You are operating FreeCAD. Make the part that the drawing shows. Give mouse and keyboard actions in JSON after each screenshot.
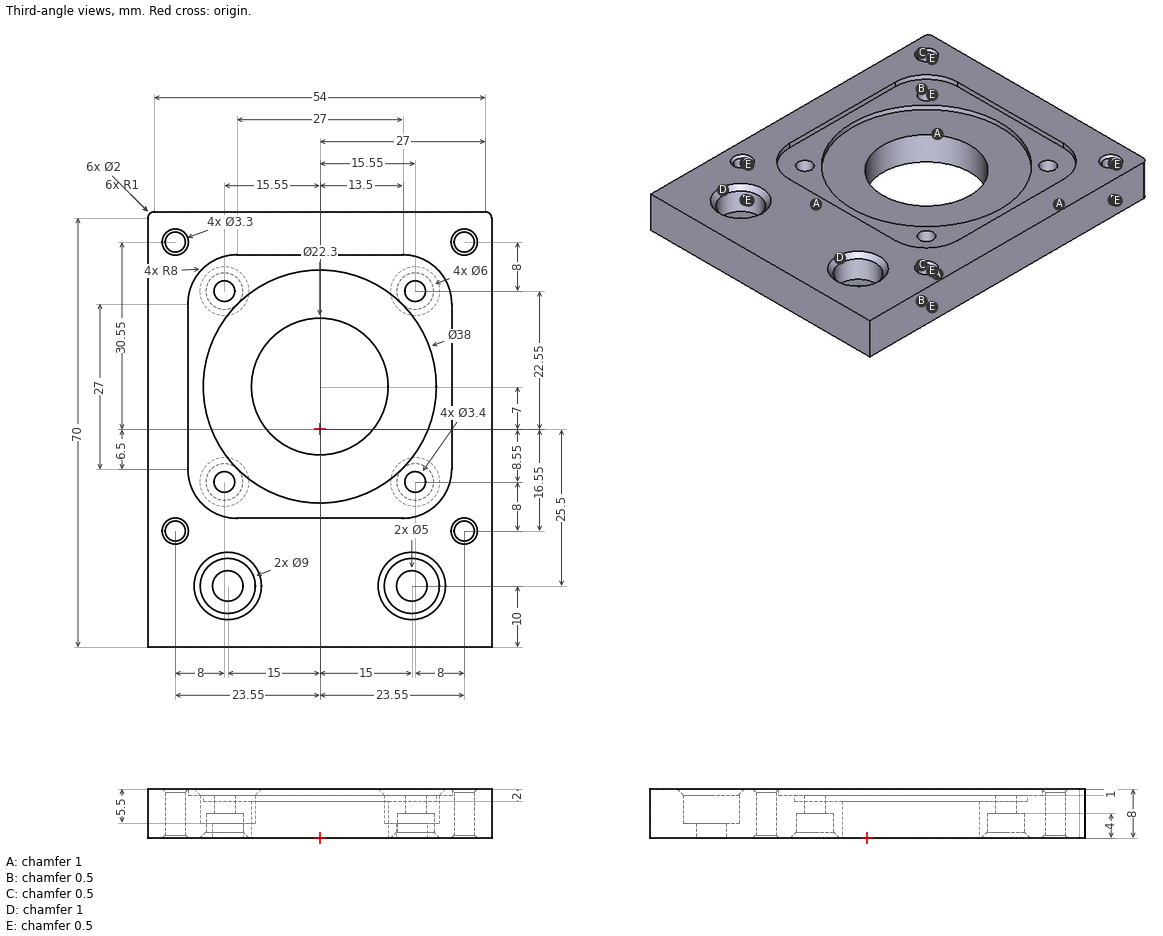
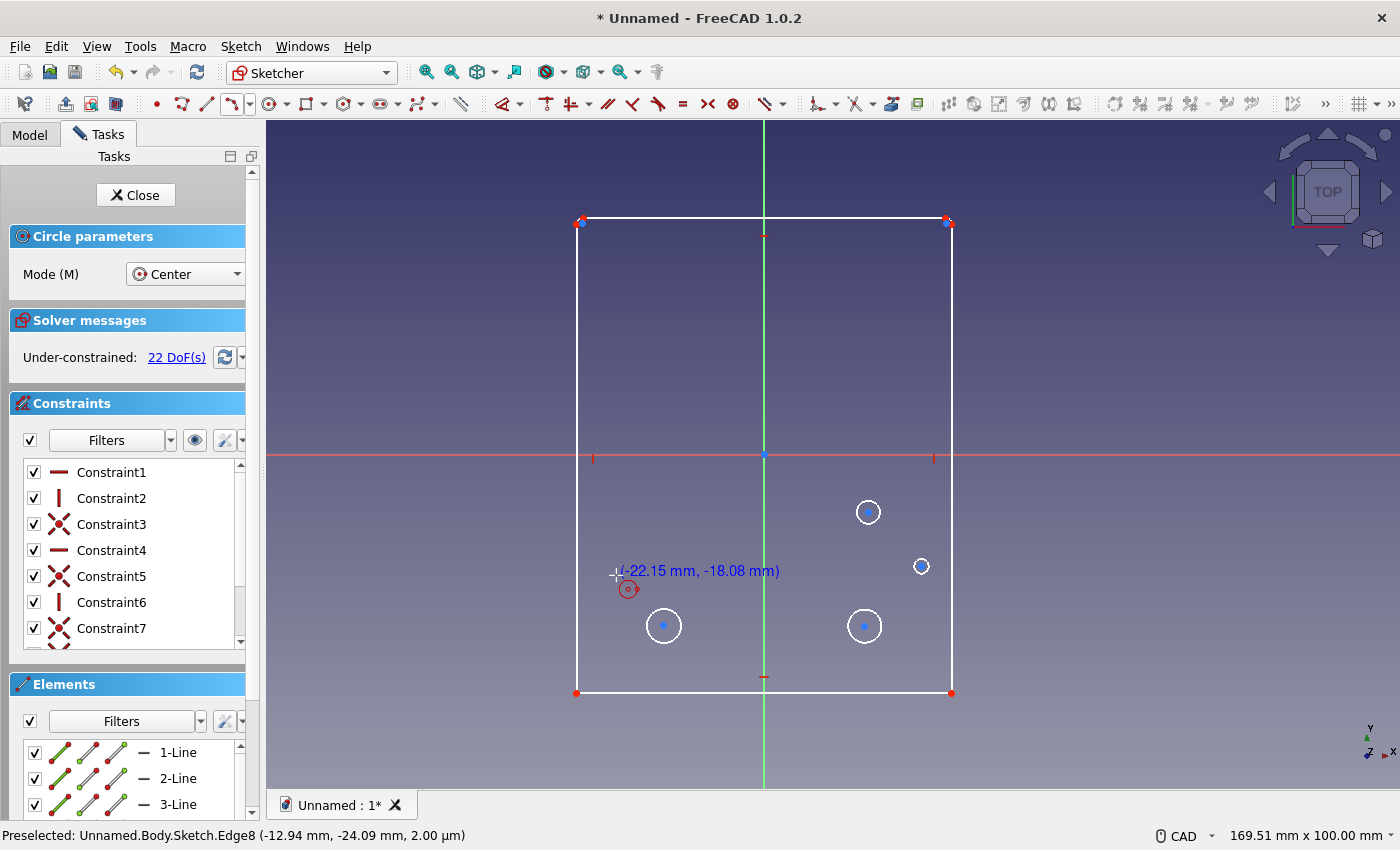
{"action": "left_click", "coordinate": [607, 566]}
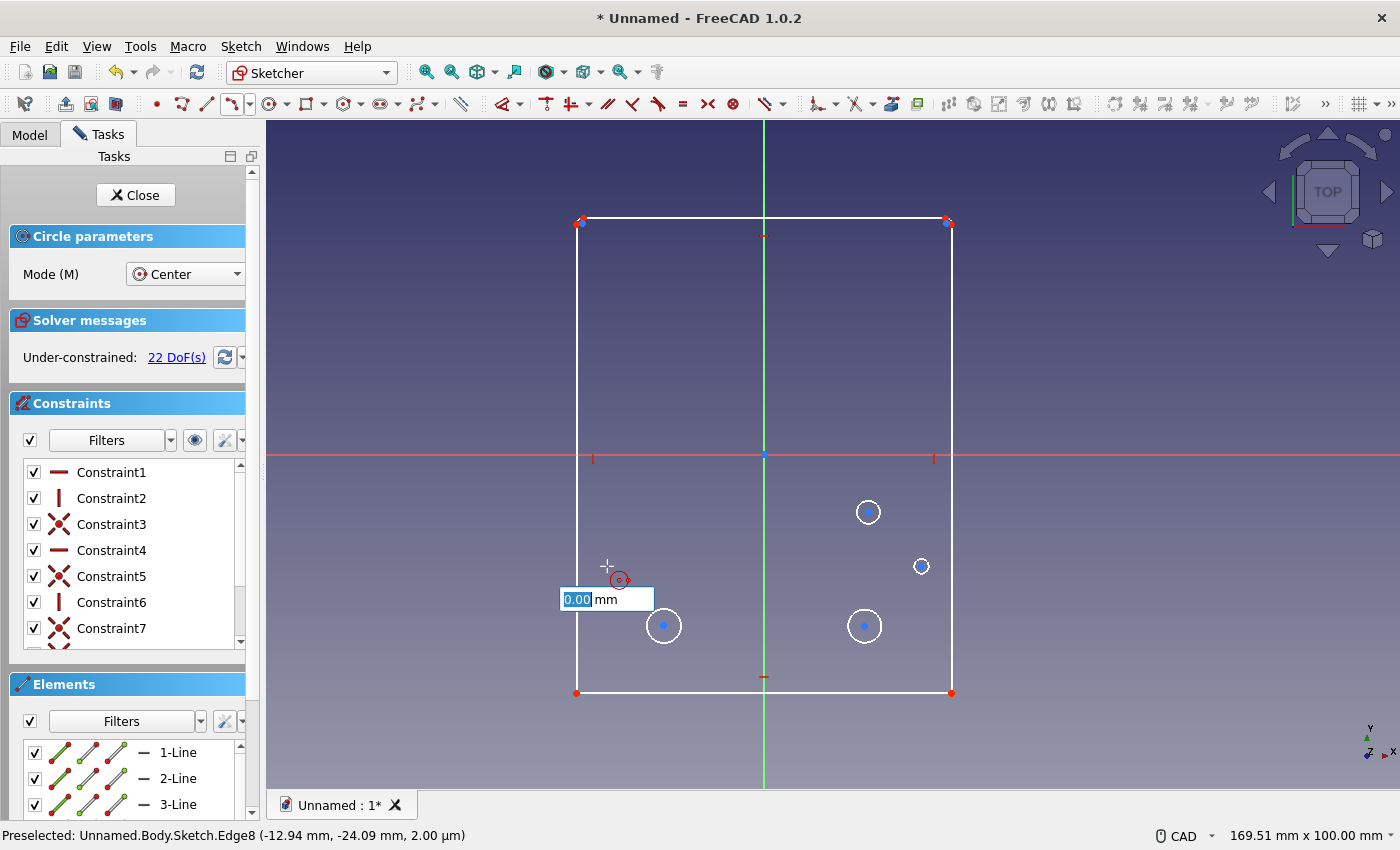
{"action": "scroll", "coordinate": [612, 561], "scroll_direction": "up", "scroll_amount": 5}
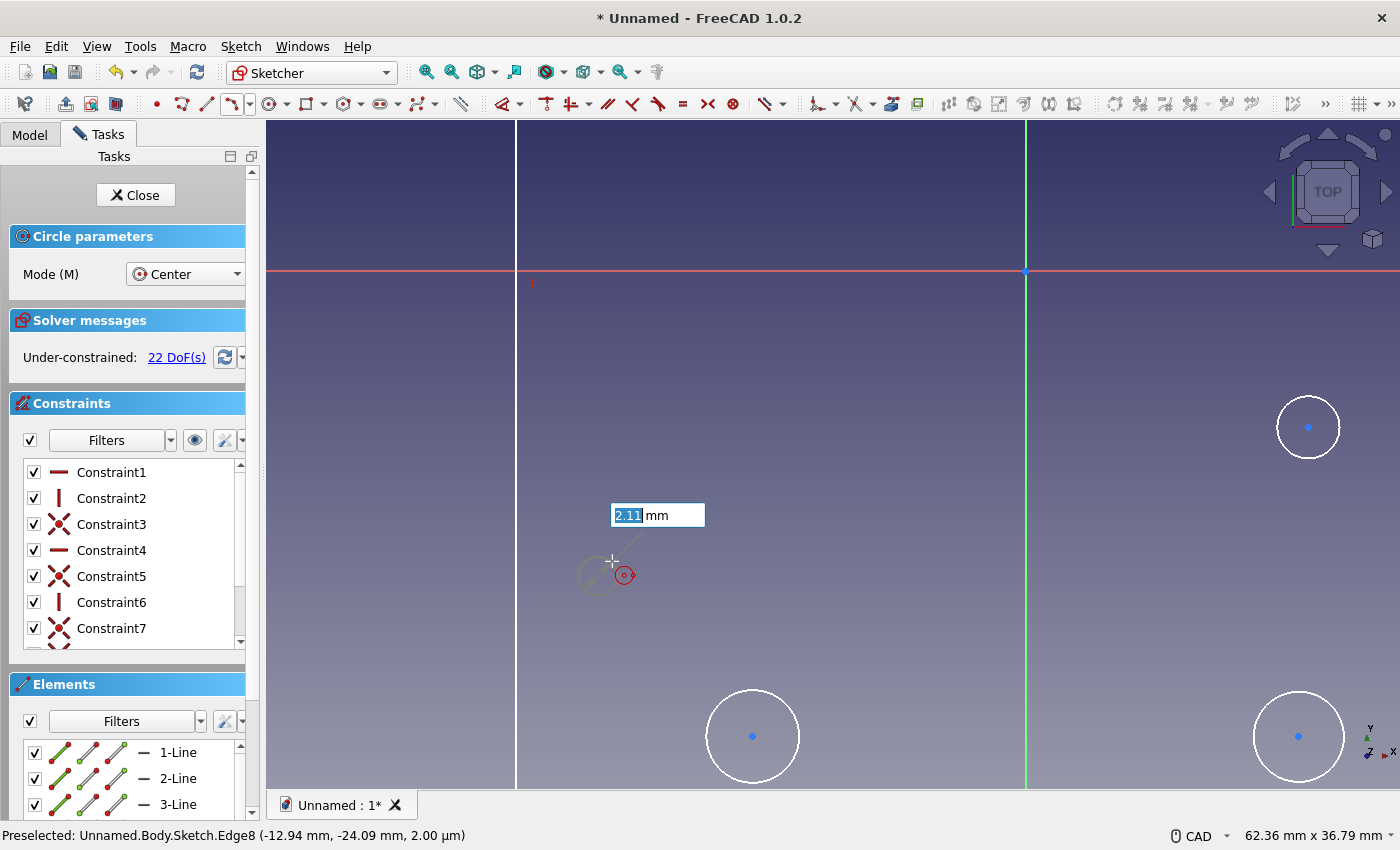
{"action": "left_click", "coordinate": [610, 559]}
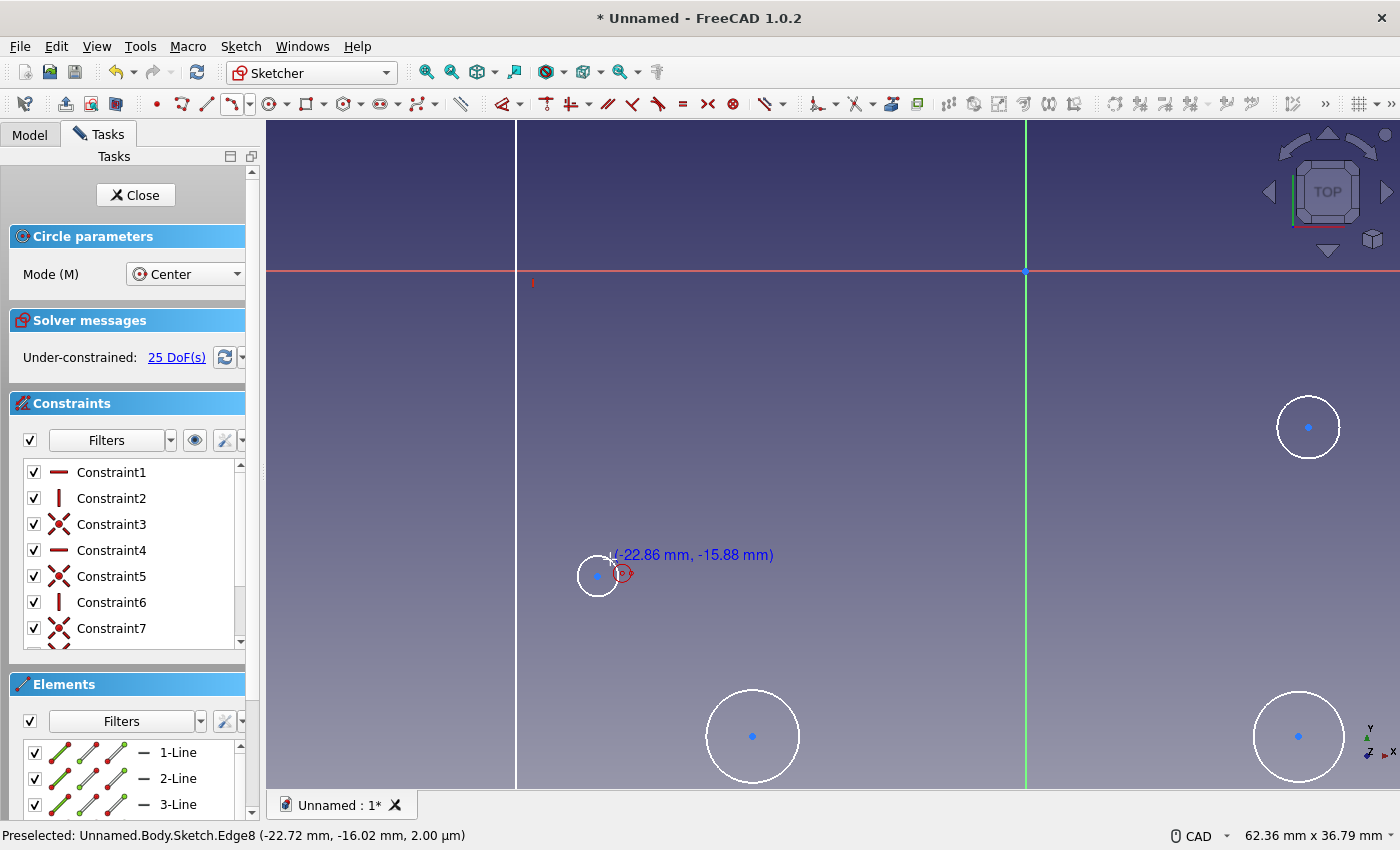
{"action": "left_click", "coordinate": [743, 427]}
{"action": "left_click", "coordinate": [765, 405]}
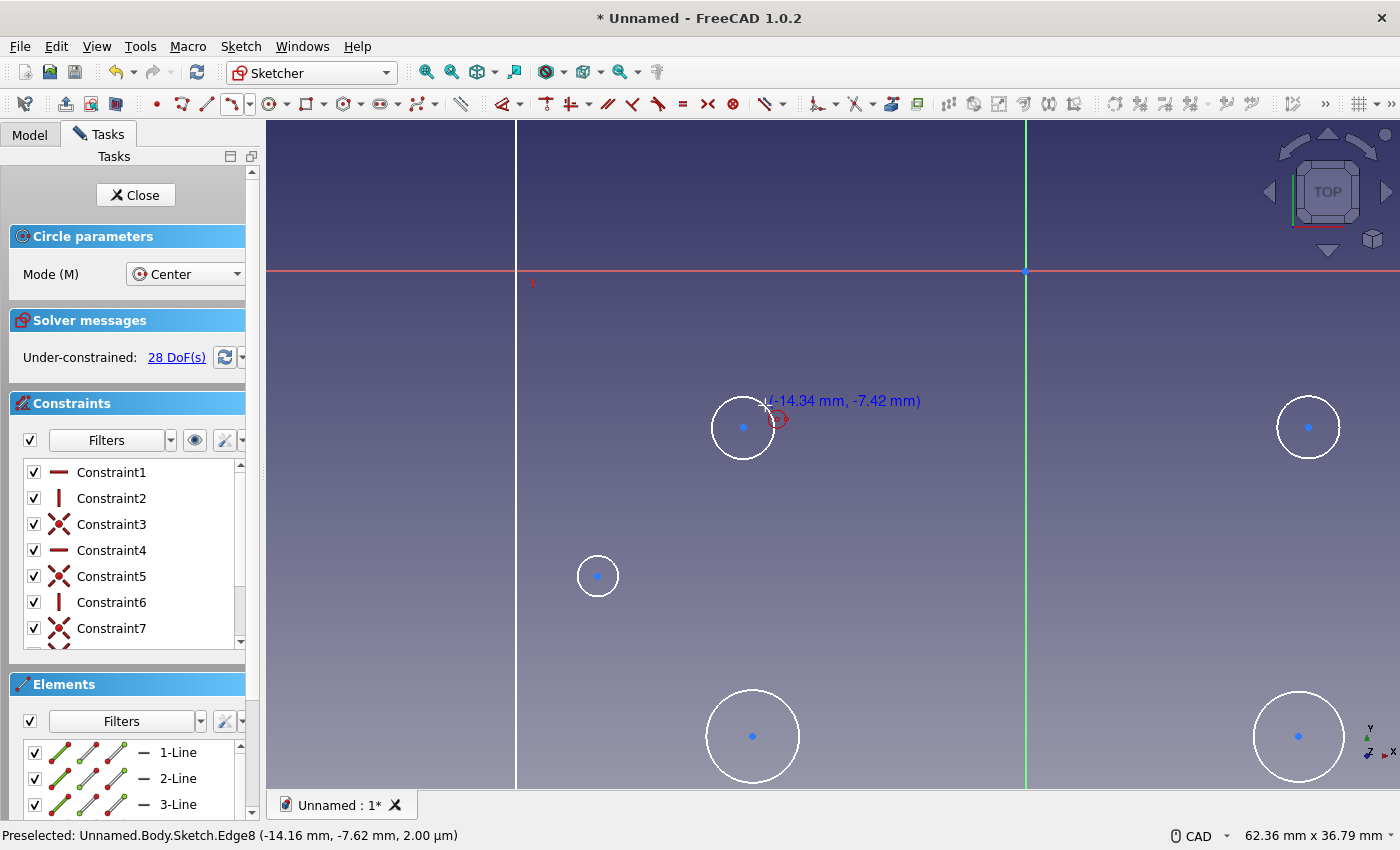
{"action": "scroll", "coordinate": [612, 561], "scroll_direction": "down", "scroll_amount": 5}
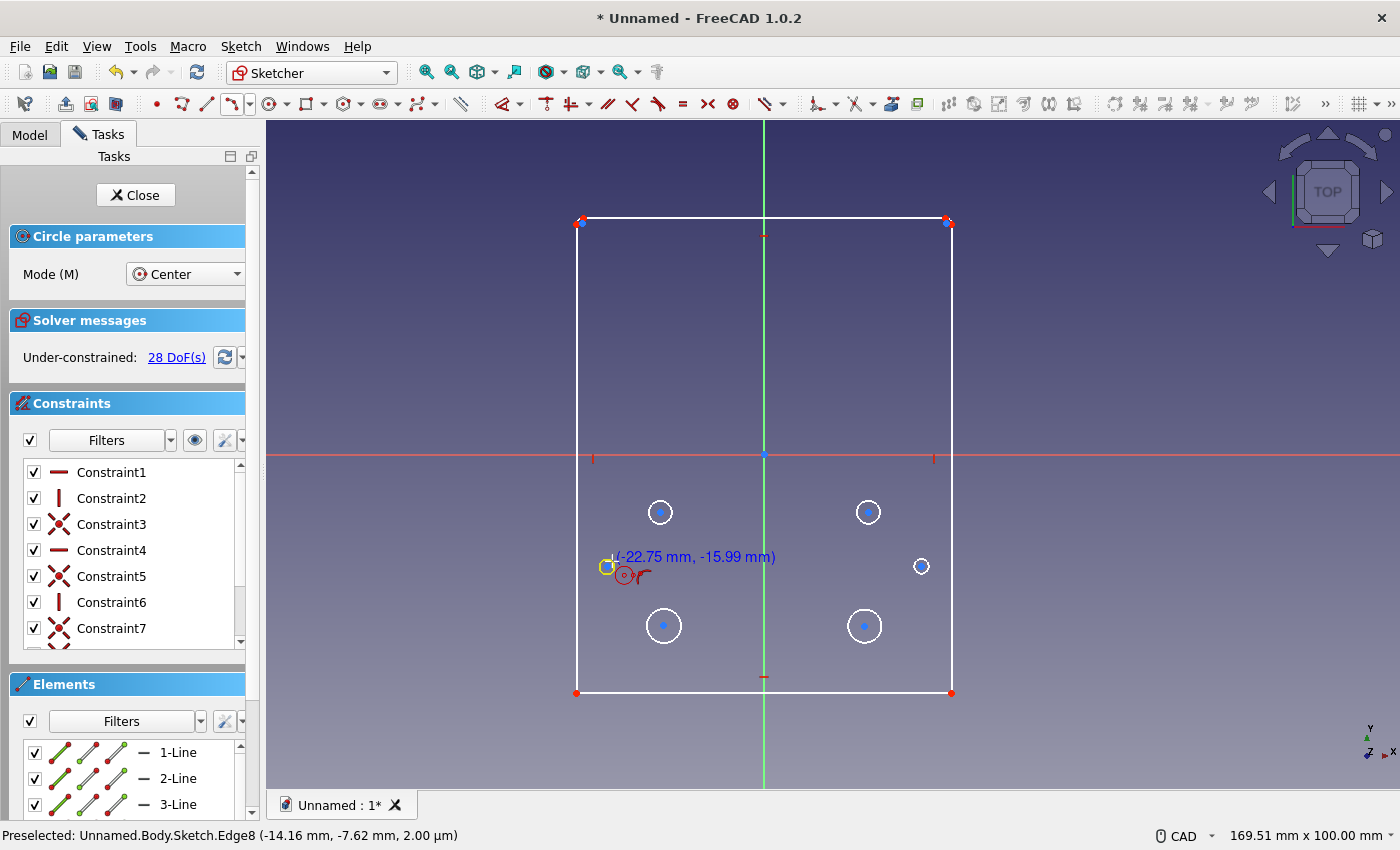
{"action": "scroll", "coordinate": [868, 304], "scroll_direction": "up", "scroll_amount": 4}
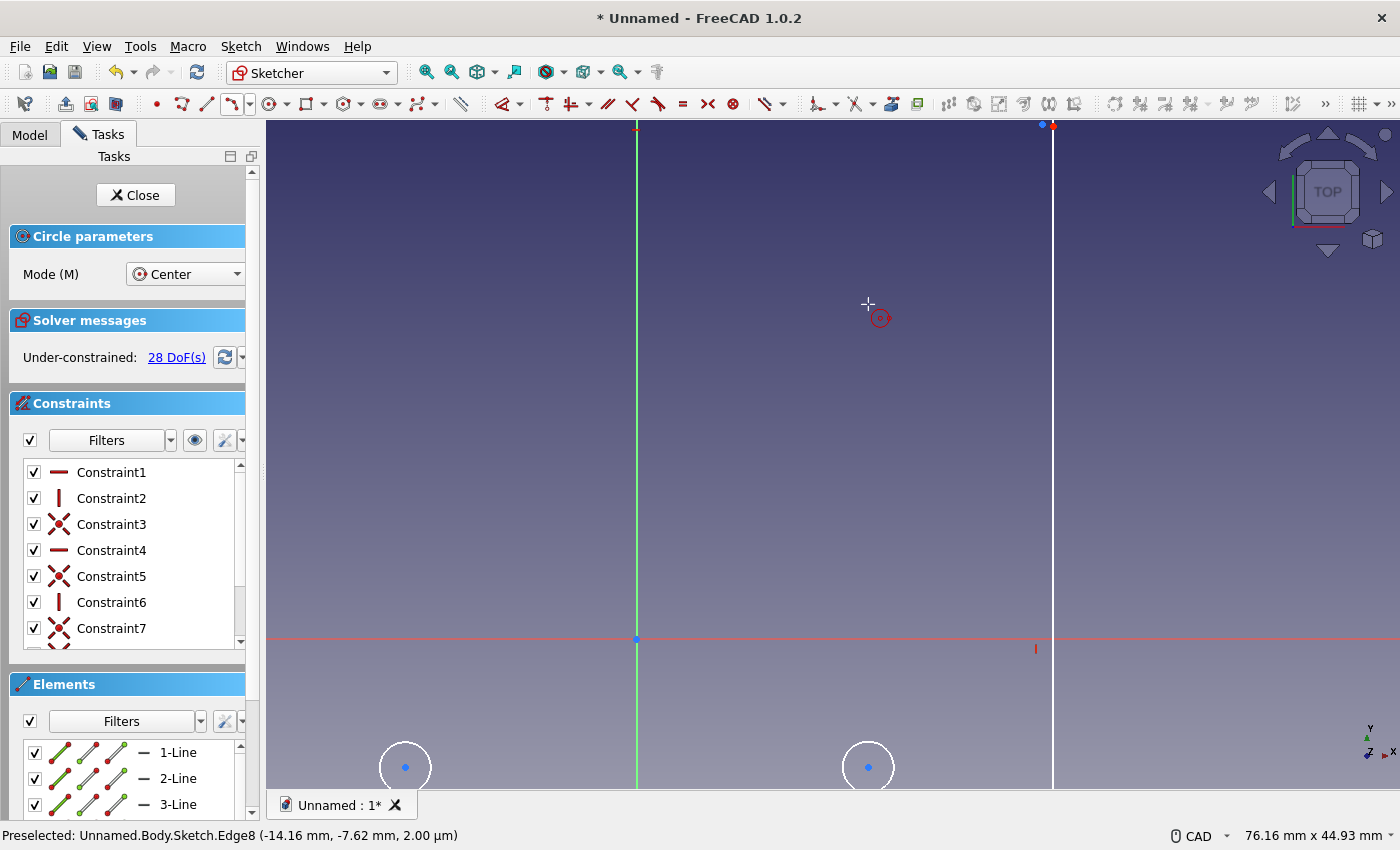
{"action": "left_click", "coordinate": [868, 303]}
{"action": "left_click", "coordinate": [886, 286]}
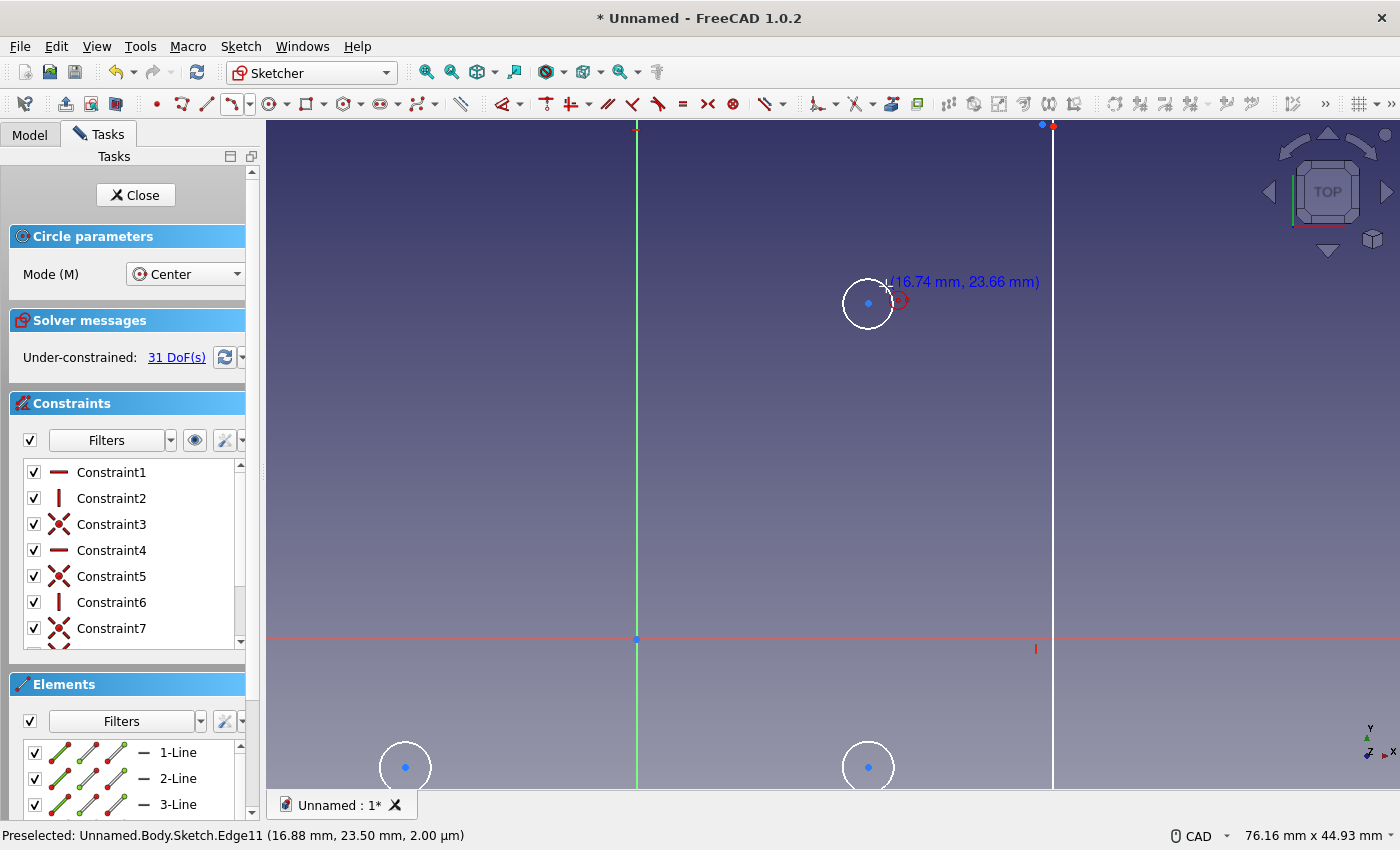
{"action": "scroll", "coordinate": [987, 184], "scroll_direction": "up", "scroll_amount": 3}